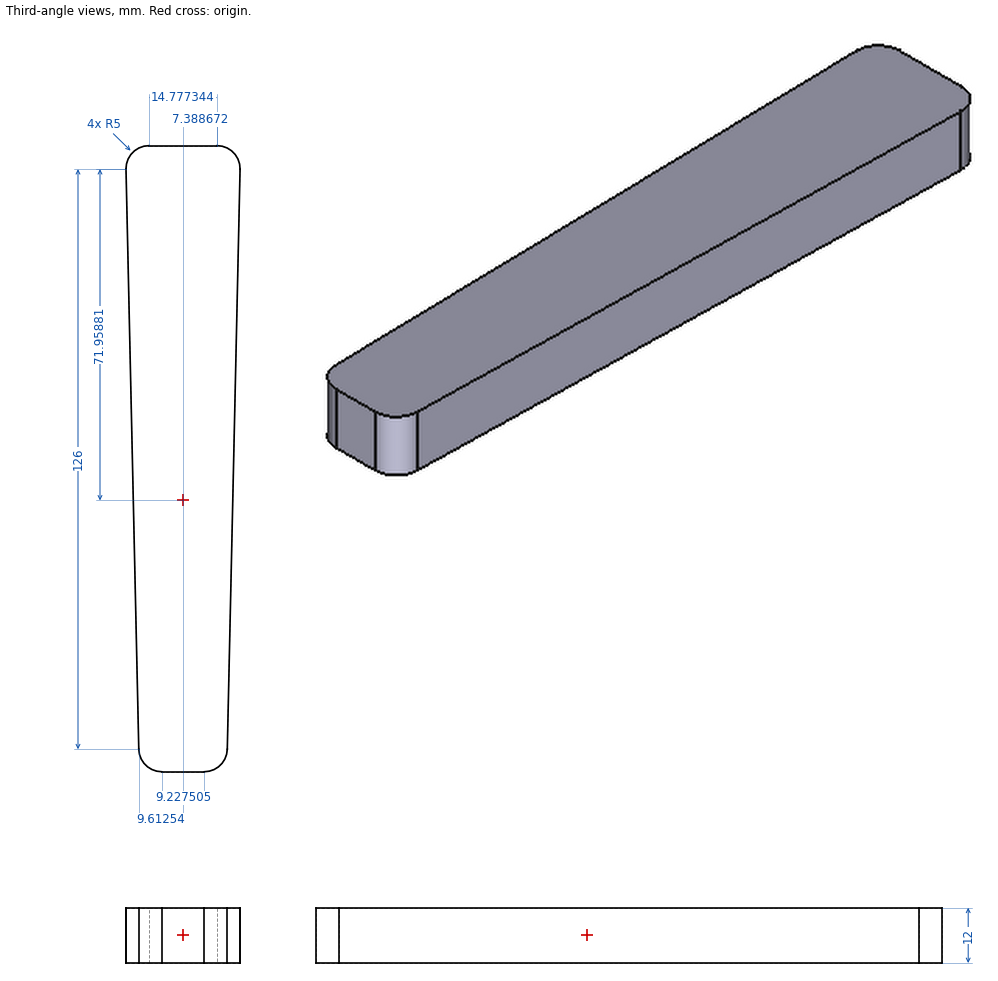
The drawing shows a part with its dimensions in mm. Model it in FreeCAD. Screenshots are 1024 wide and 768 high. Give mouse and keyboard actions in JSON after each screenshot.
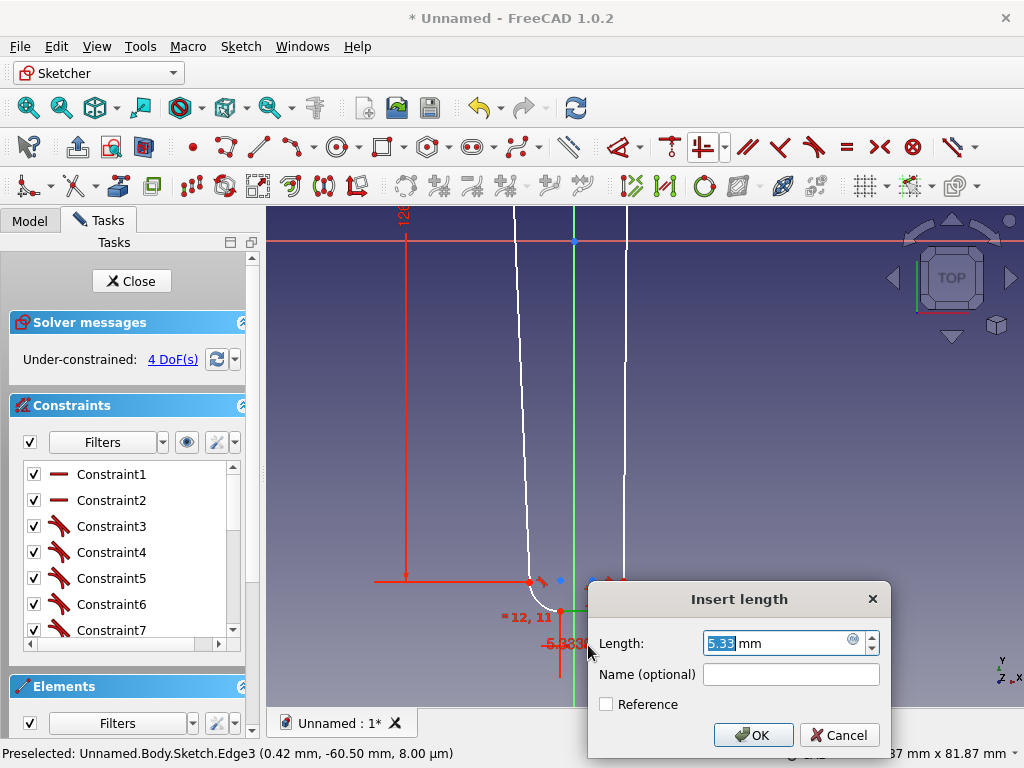
{"action": "type", "text": "9.227505"}
{"action": "key", "text": "Return"}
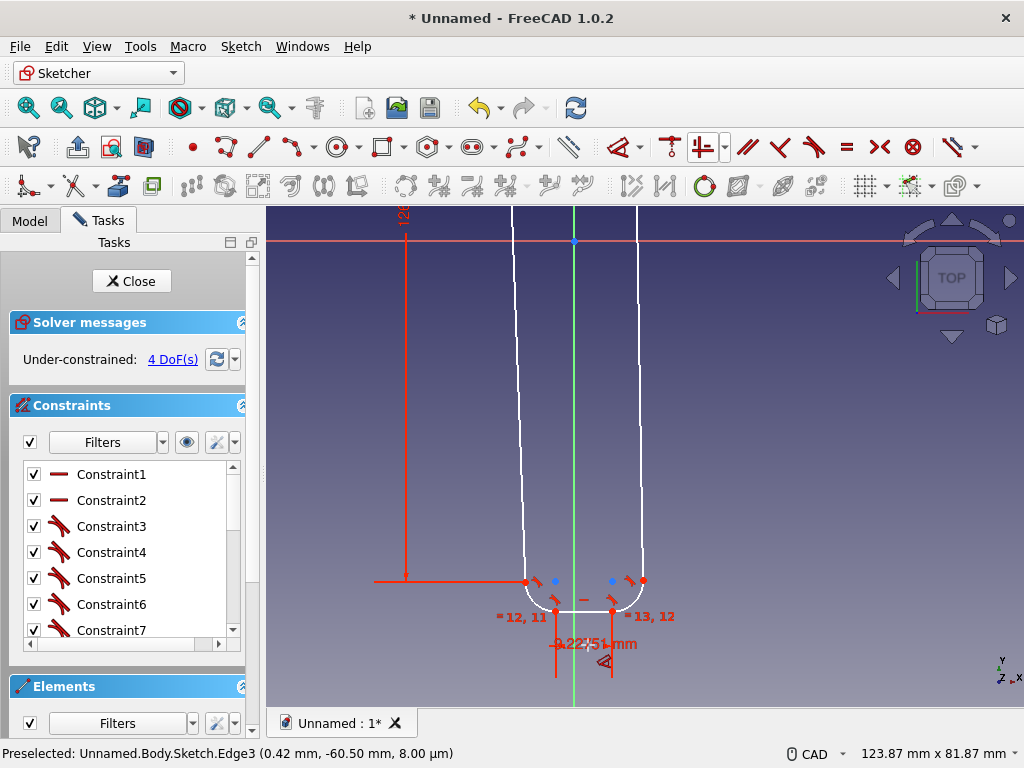
{"action": "left_click", "coordinate": [525, 582]}
{"action": "left_click", "coordinate": [539, 616]}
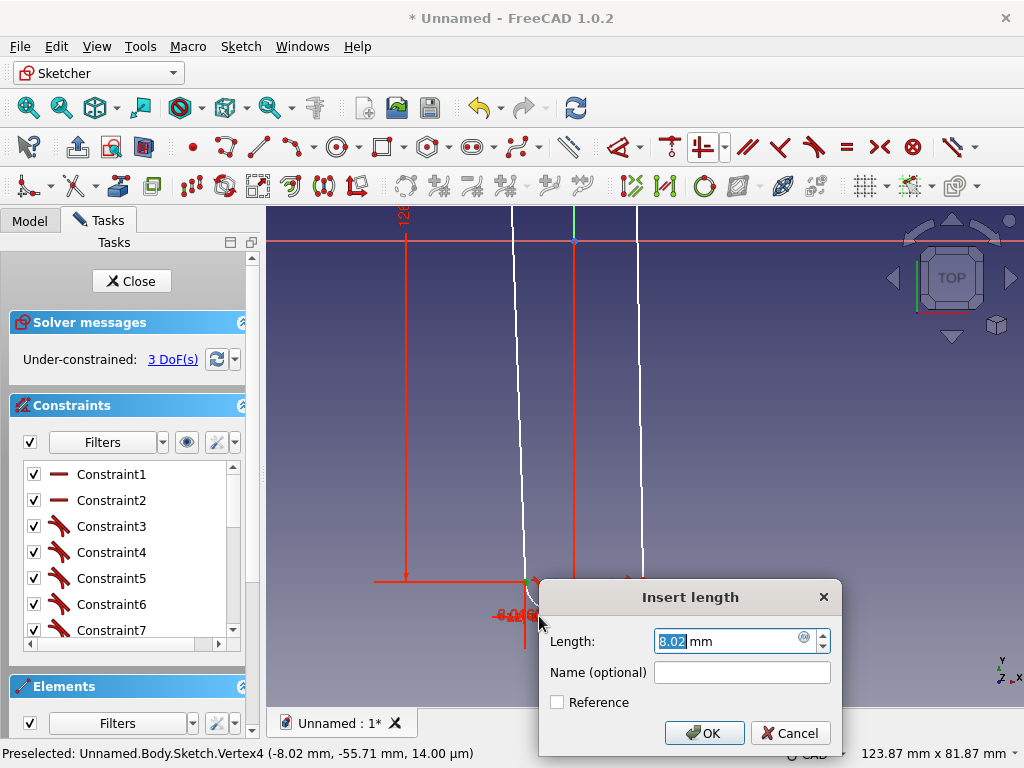
{"action": "type", "text": "9.61254"}
{"action": "key", "text": "Return"}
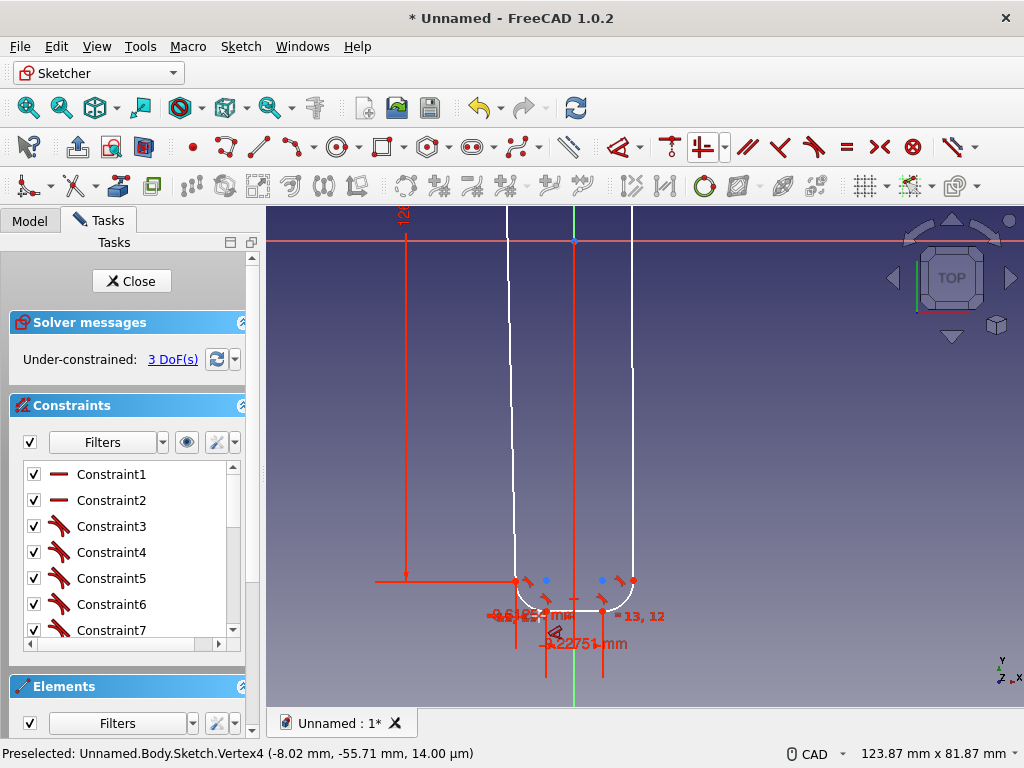
{"action": "scroll", "coordinate": [578, 614], "scroll_direction": "down", "scroll_amount": 5}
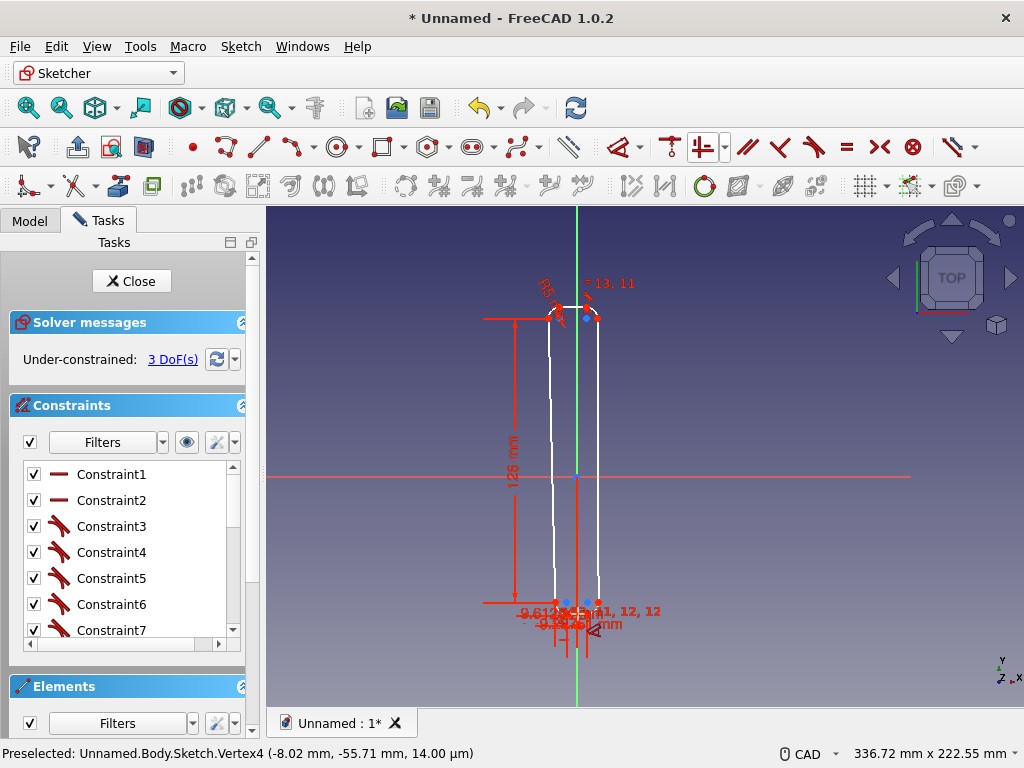
{"action": "scroll", "coordinate": [578, 307], "scroll_direction": "up", "scroll_amount": 3}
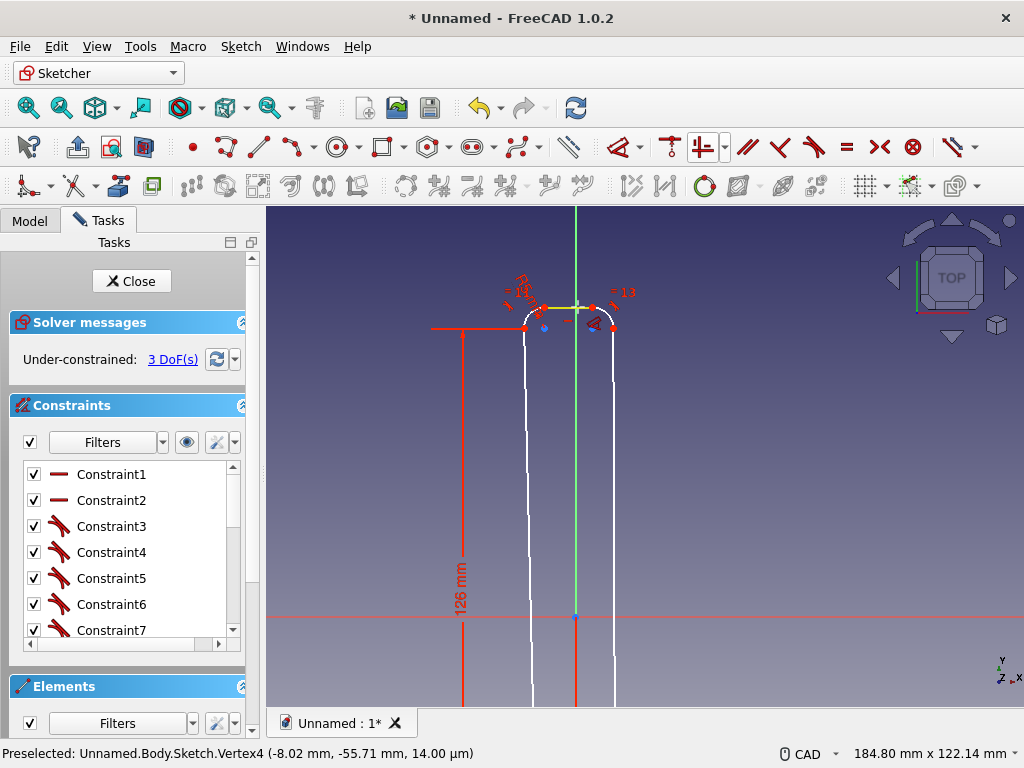
{"action": "left_click", "coordinate": [578, 308]}
{"action": "left_click", "coordinate": [558, 342]}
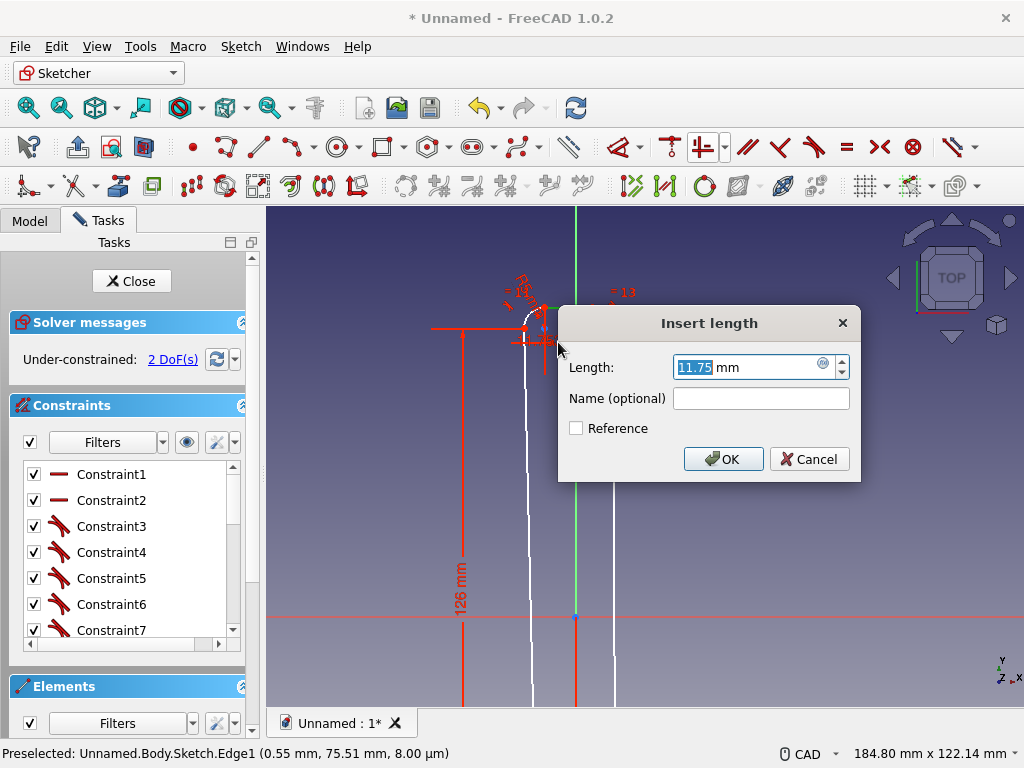
{"action": "type", "text": "14.777344"}
{"action": "key", "text": "Return"}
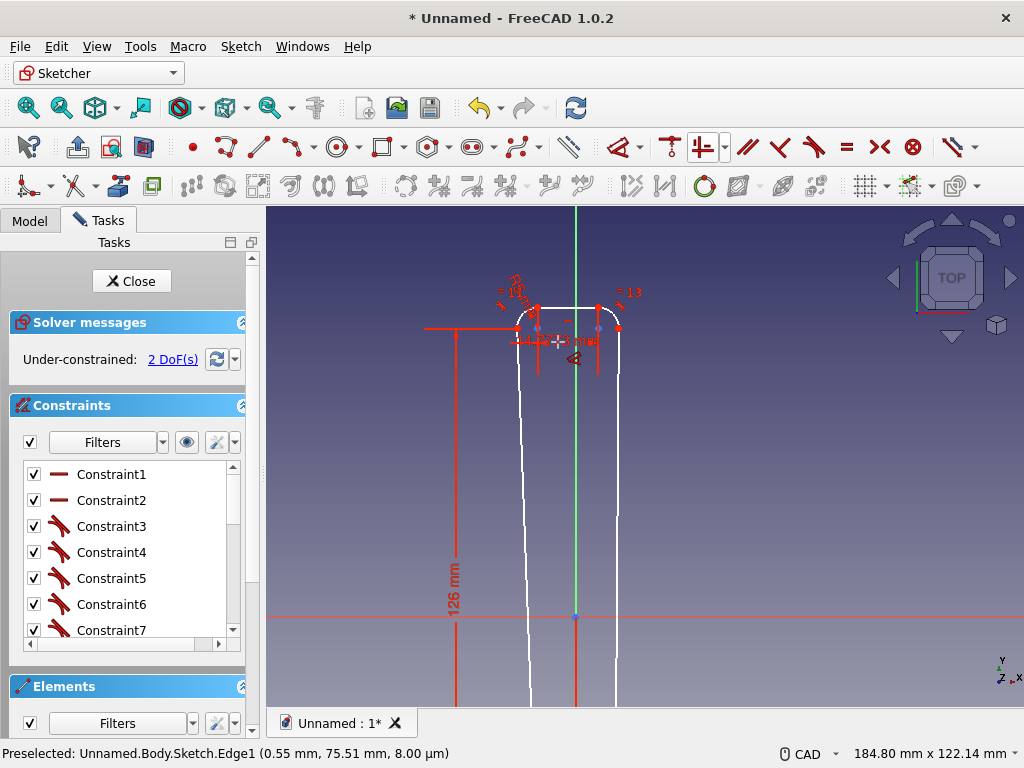
{"action": "scroll", "coordinate": [598, 308], "scroll_direction": "up", "scroll_amount": 2}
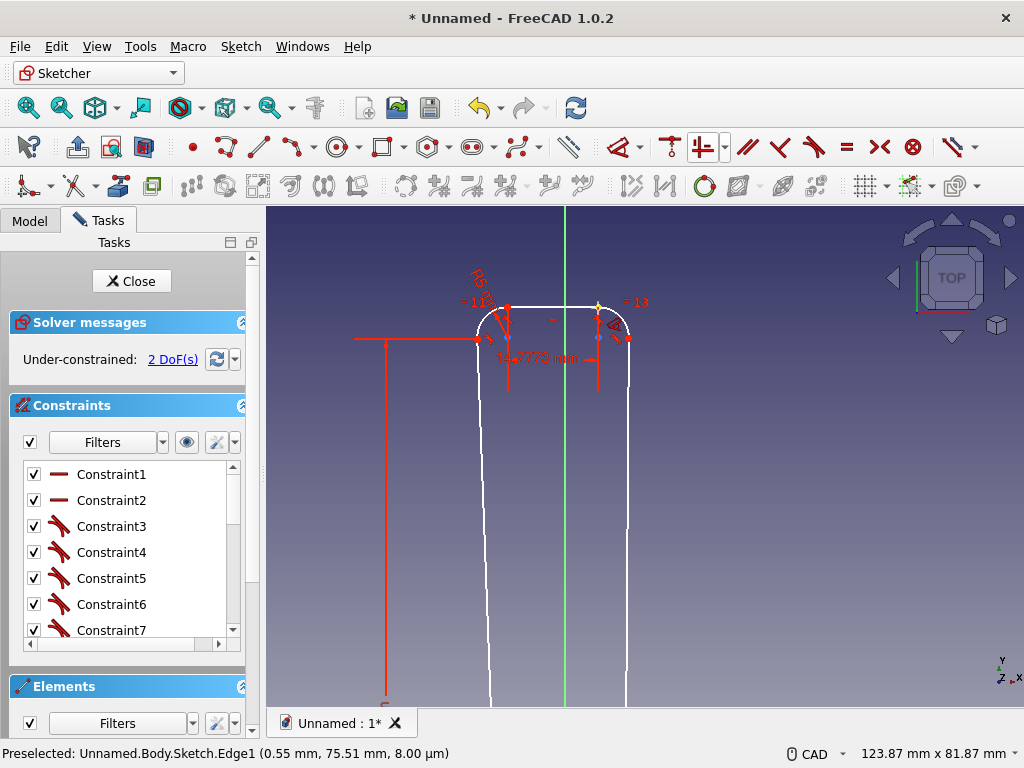
{"action": "left_click", "coordinate": [598, 307]}
{"action": "left_click", "coordinate": [581, 273]}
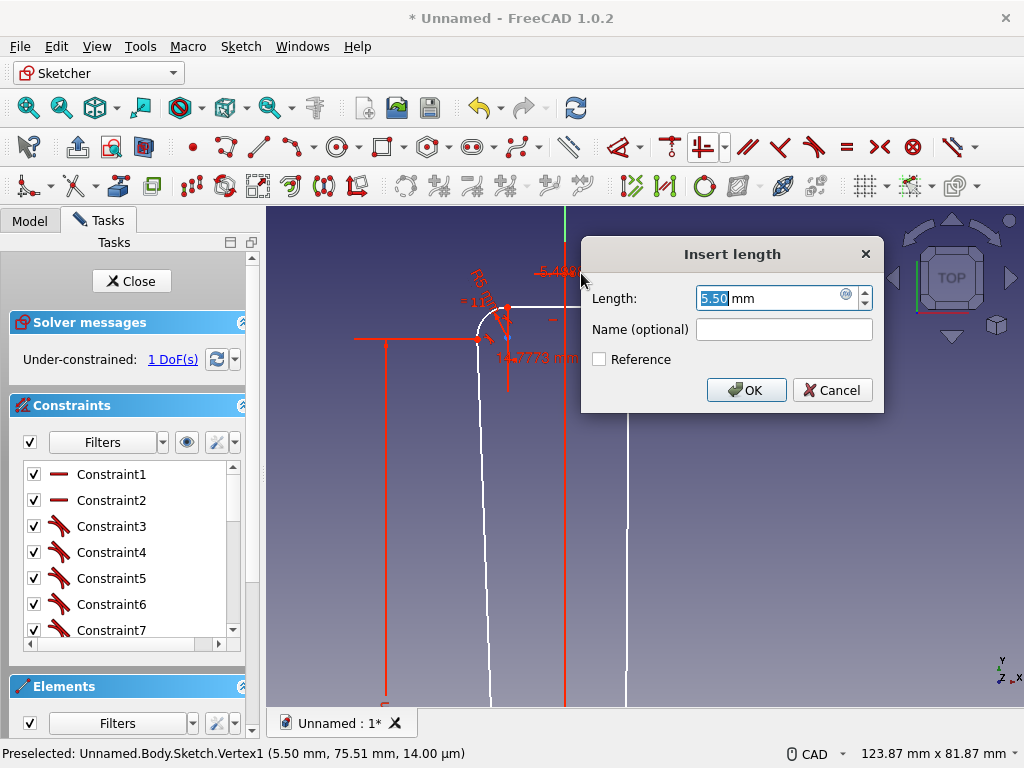
{"action": "type", "text": "7.388672"}
{"action": "key", "text": "Return"}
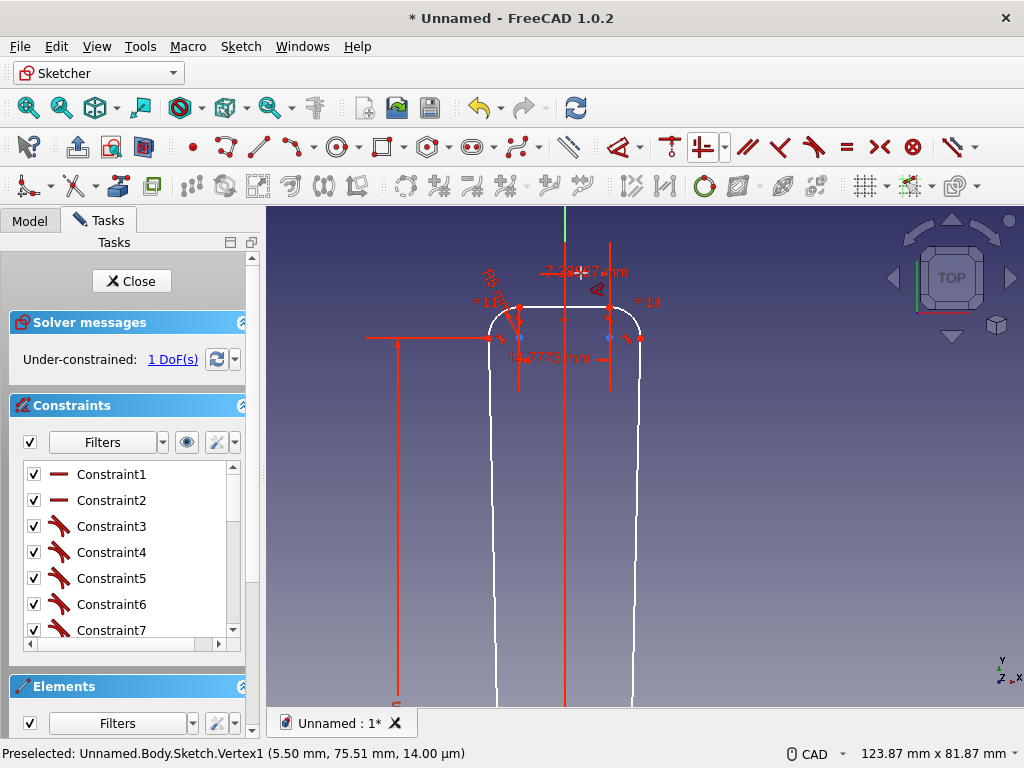
{"action": "left_click", "coordinate": [489, 338]}
{"action": "left_click", "coordinate": [455, 509]}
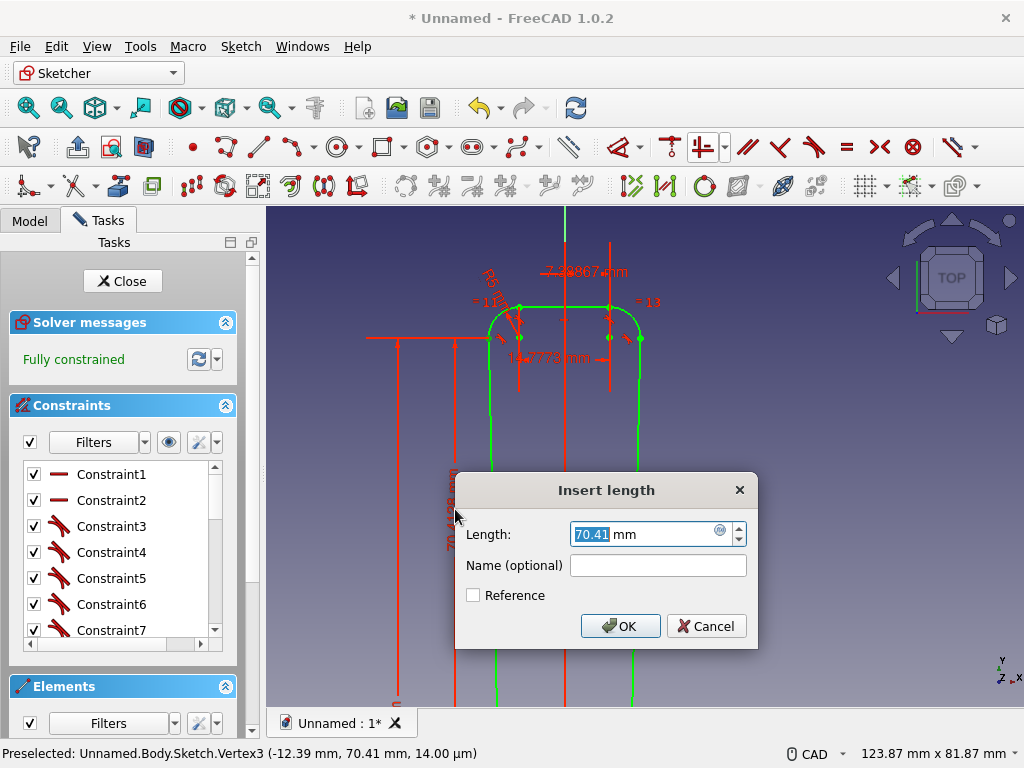
{"action": "type", "text": "71.95881"}
{"action": "key", "text": "Return"}
{"action": "key", "text": "Escape"}